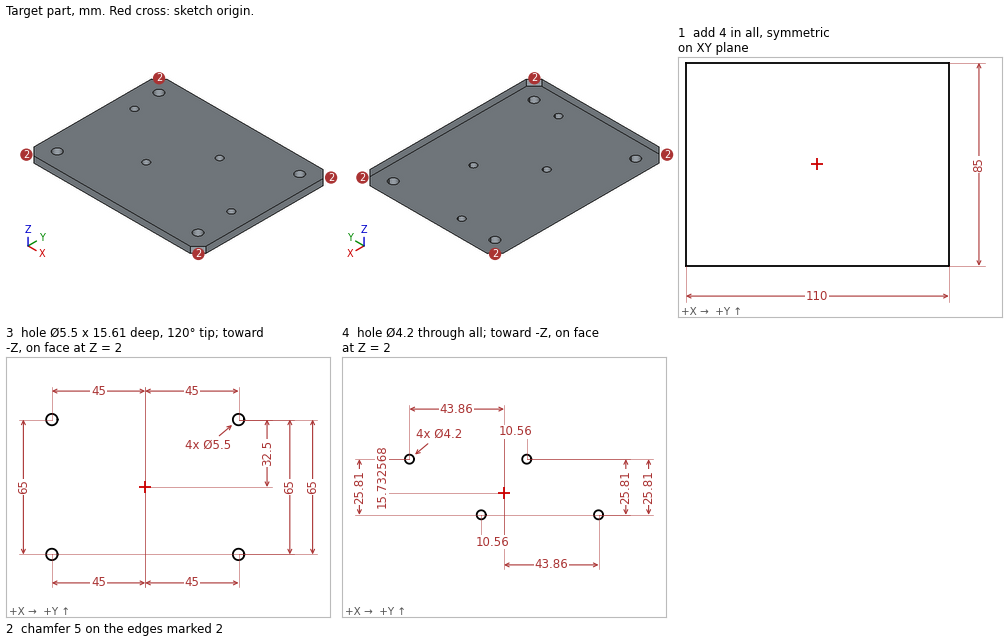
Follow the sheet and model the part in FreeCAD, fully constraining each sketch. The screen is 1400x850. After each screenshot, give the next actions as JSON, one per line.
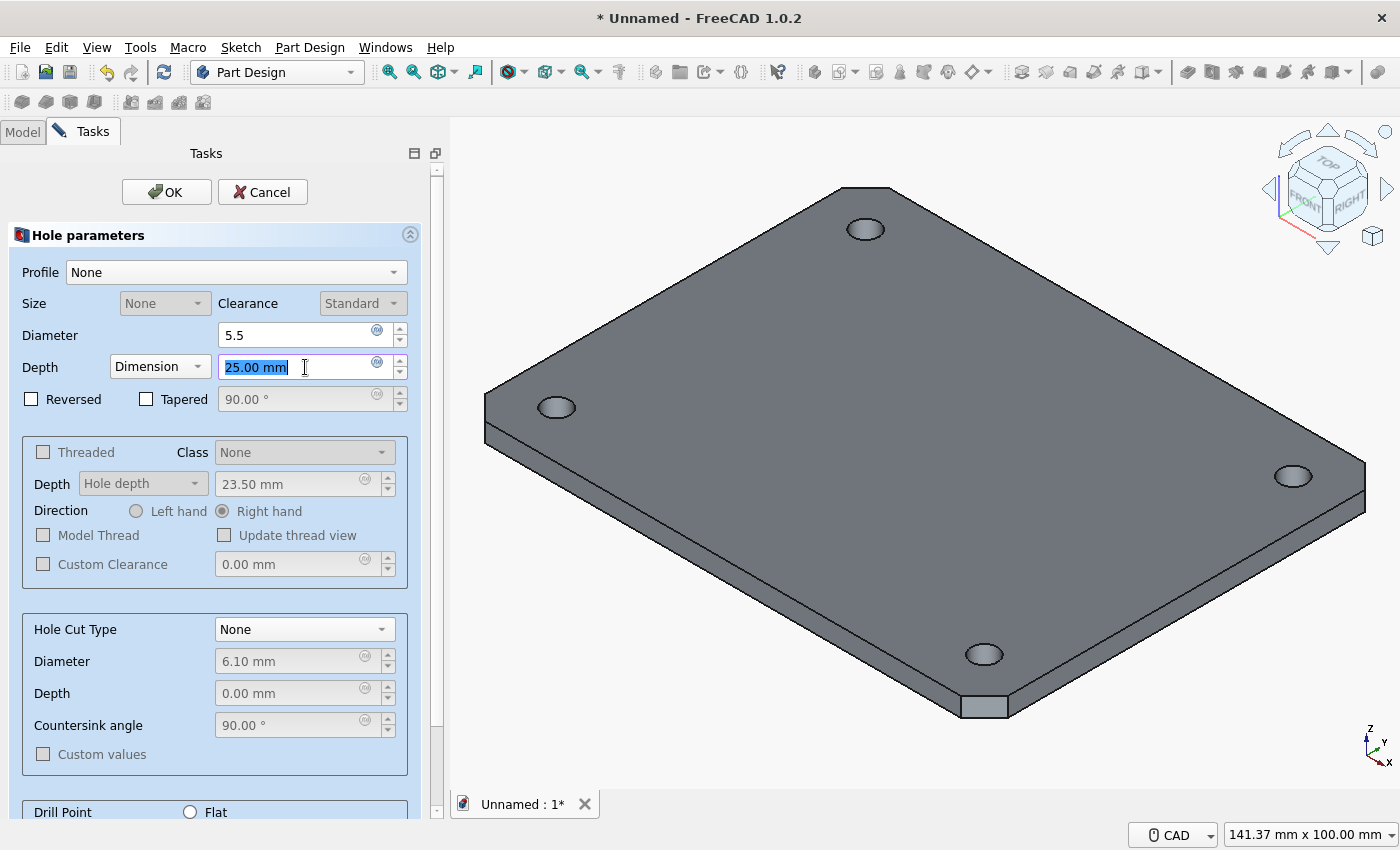
{"action": "type", "text": "15.61"}
{"action": "key", "text": "Tab"}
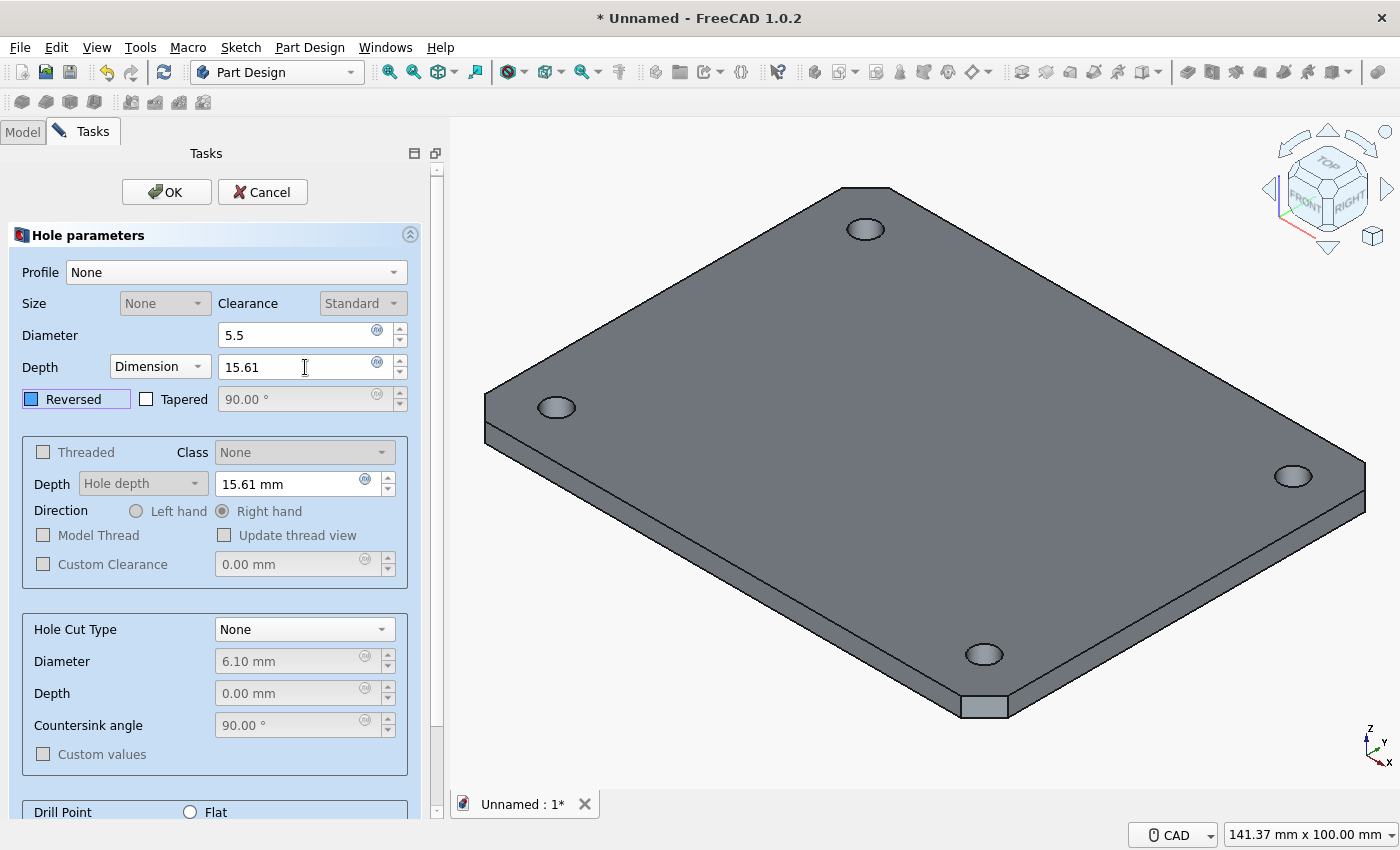
{"action": "scroll", "coordinate": [437, 490], "scroll_direction": "down", "scroll_amount": 2}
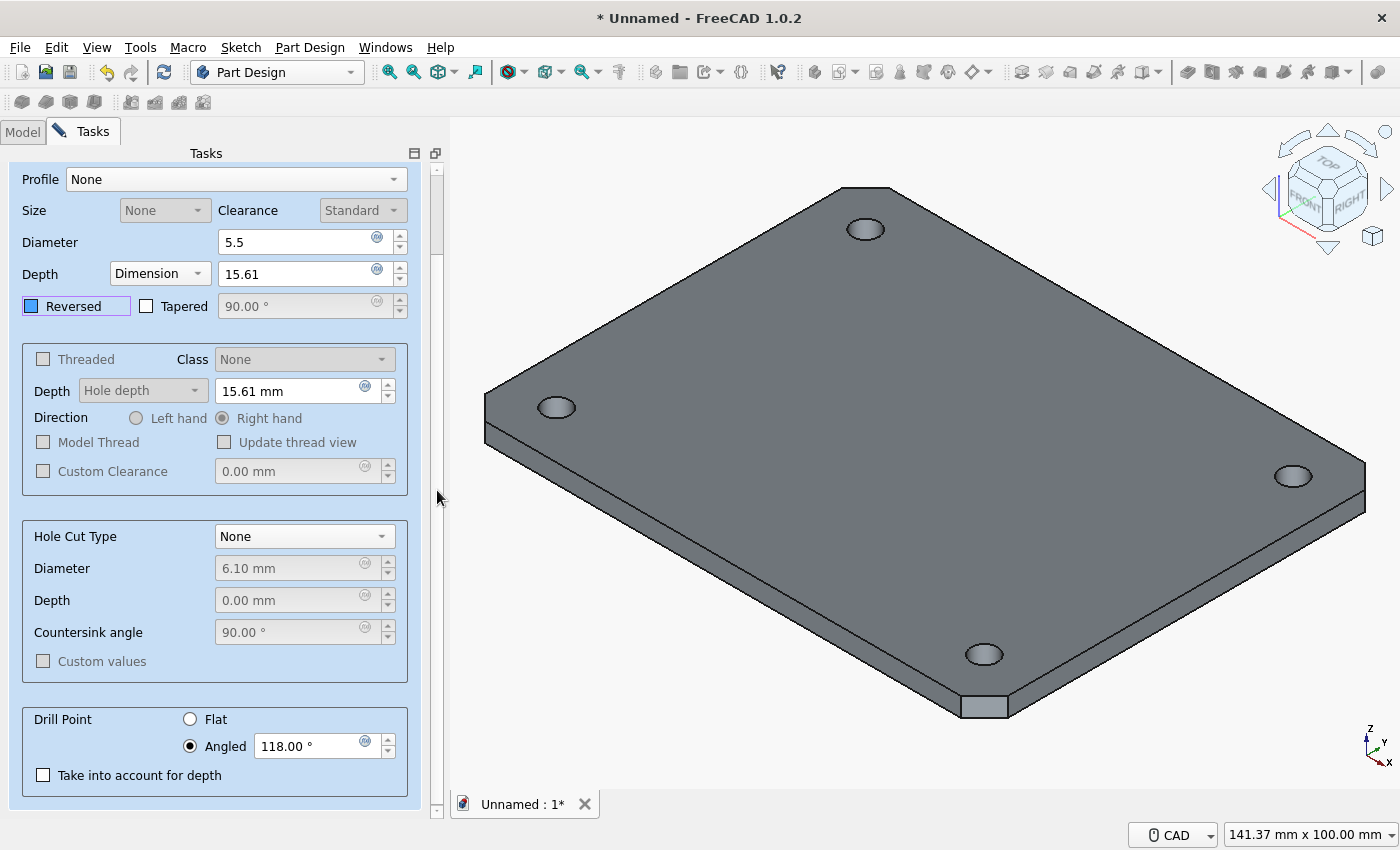
{"action": "triple_click", "coordinate": [317, 746]}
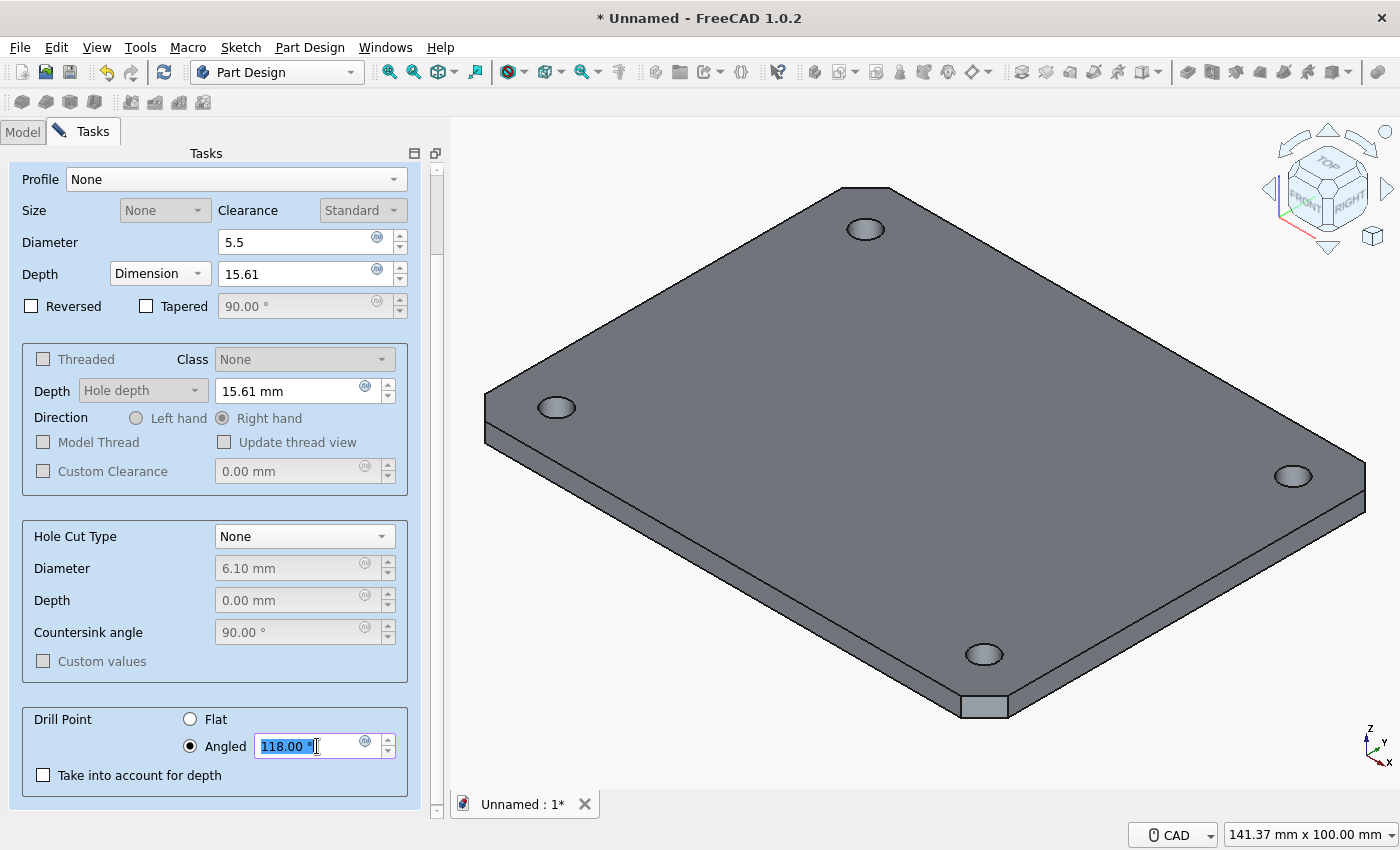
{"action": "type", "text": "120"}
{"action": "key", "text": "Tab"}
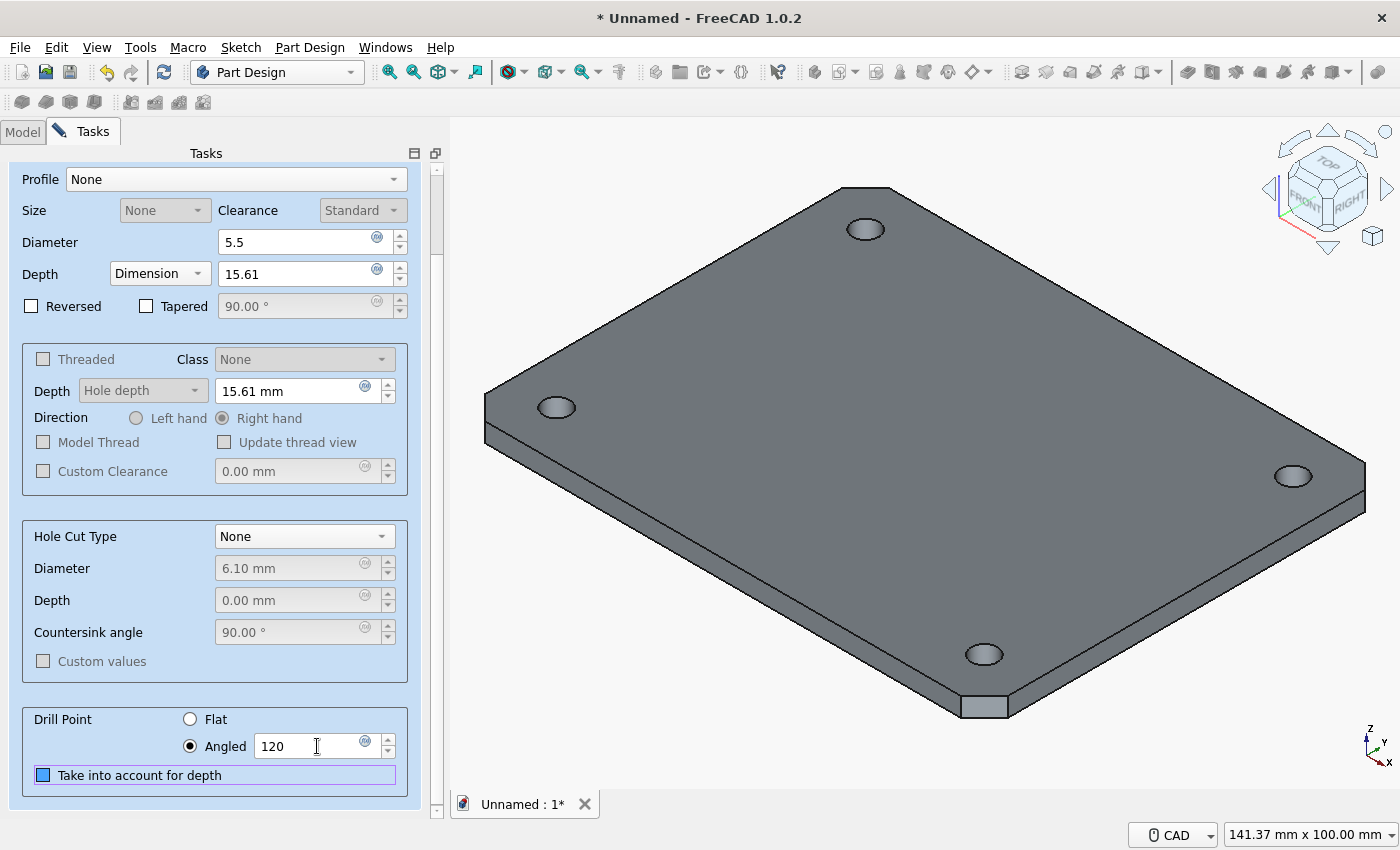
{"action": "scroll", "coordinate": [437, 490], "scroll_direction": "up", "scroll_amount": 3}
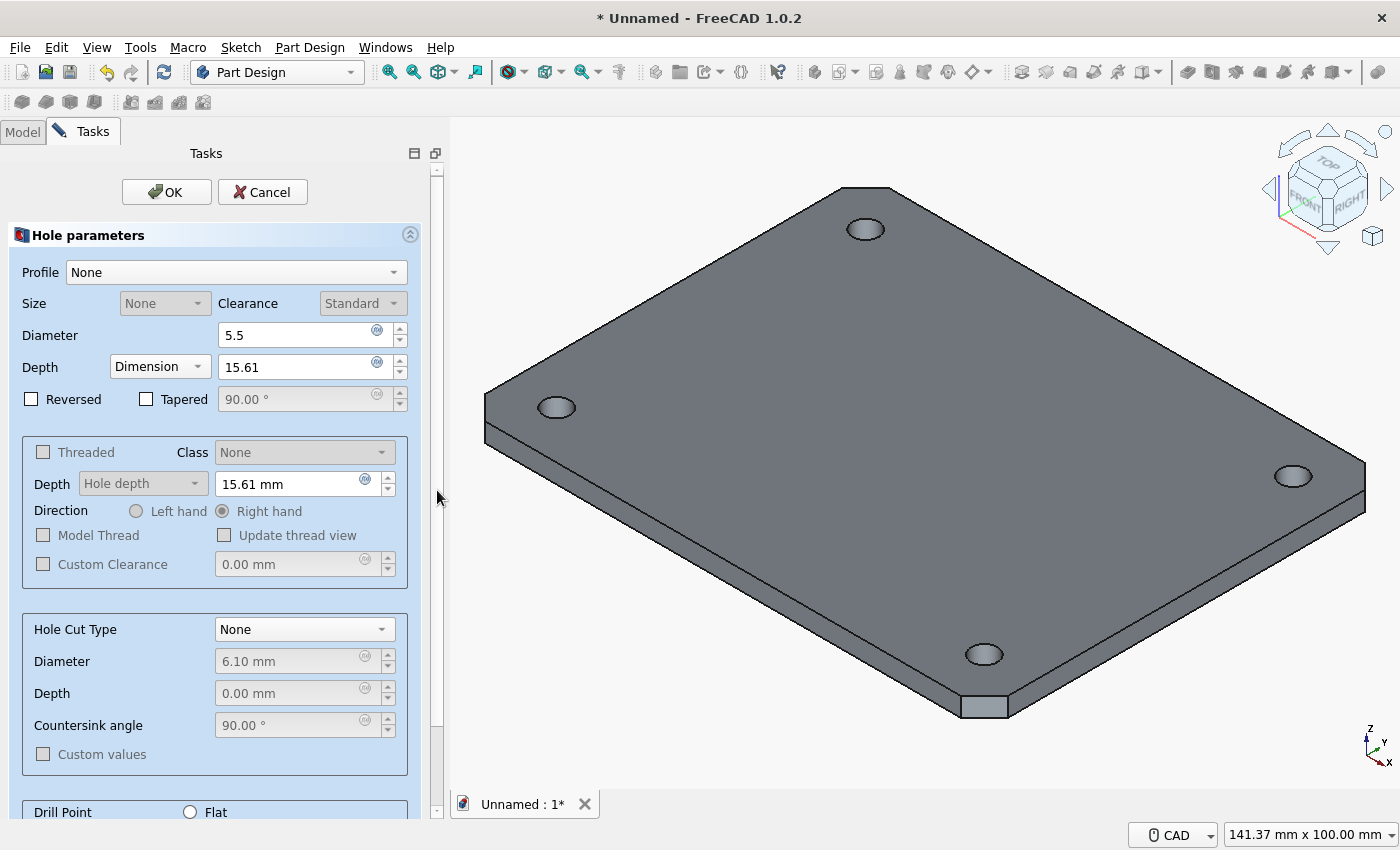
{"action": "left_click", "coordinate": [167, 192]}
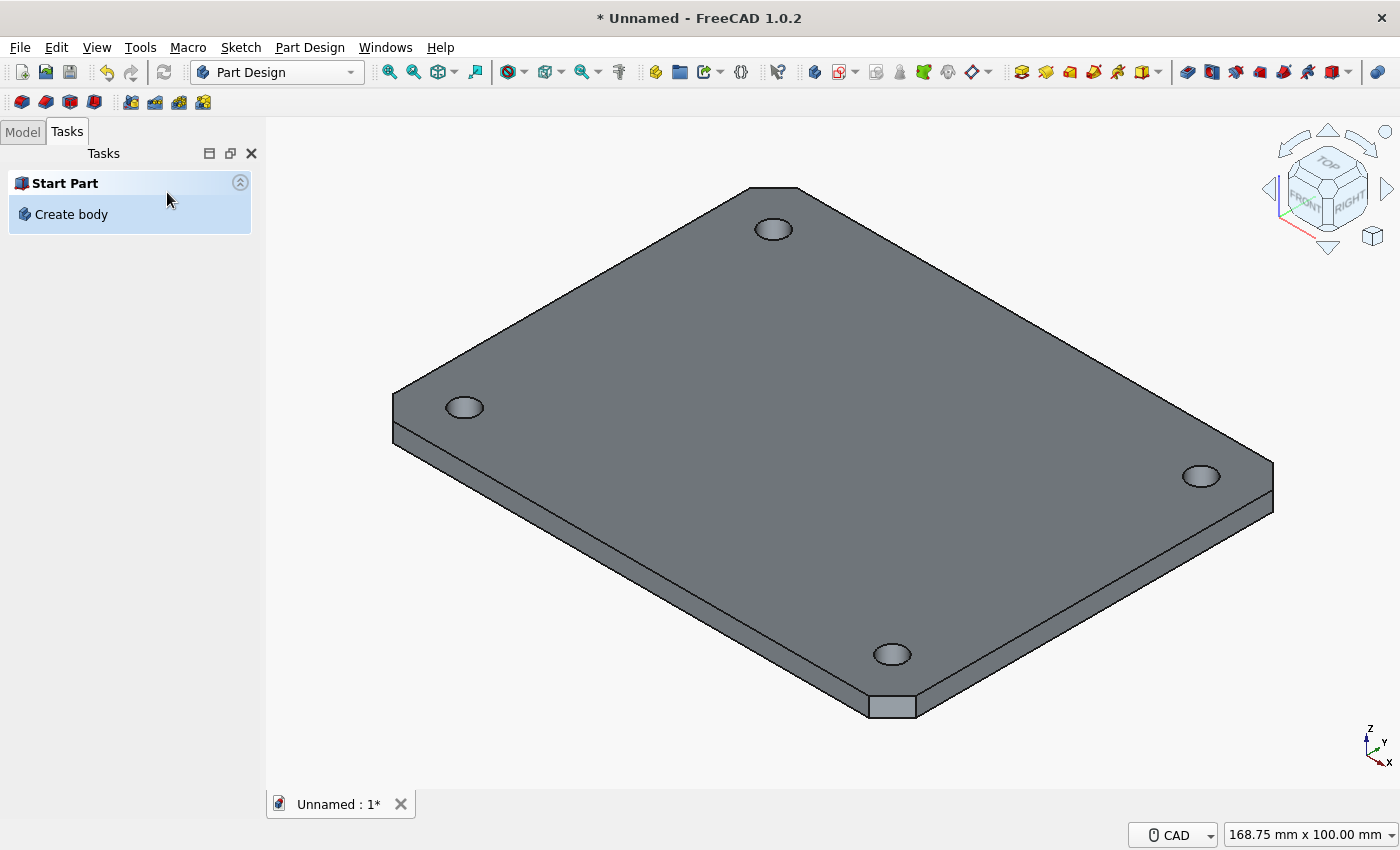
{"action": "left_click", "coordinate": [833, 441]}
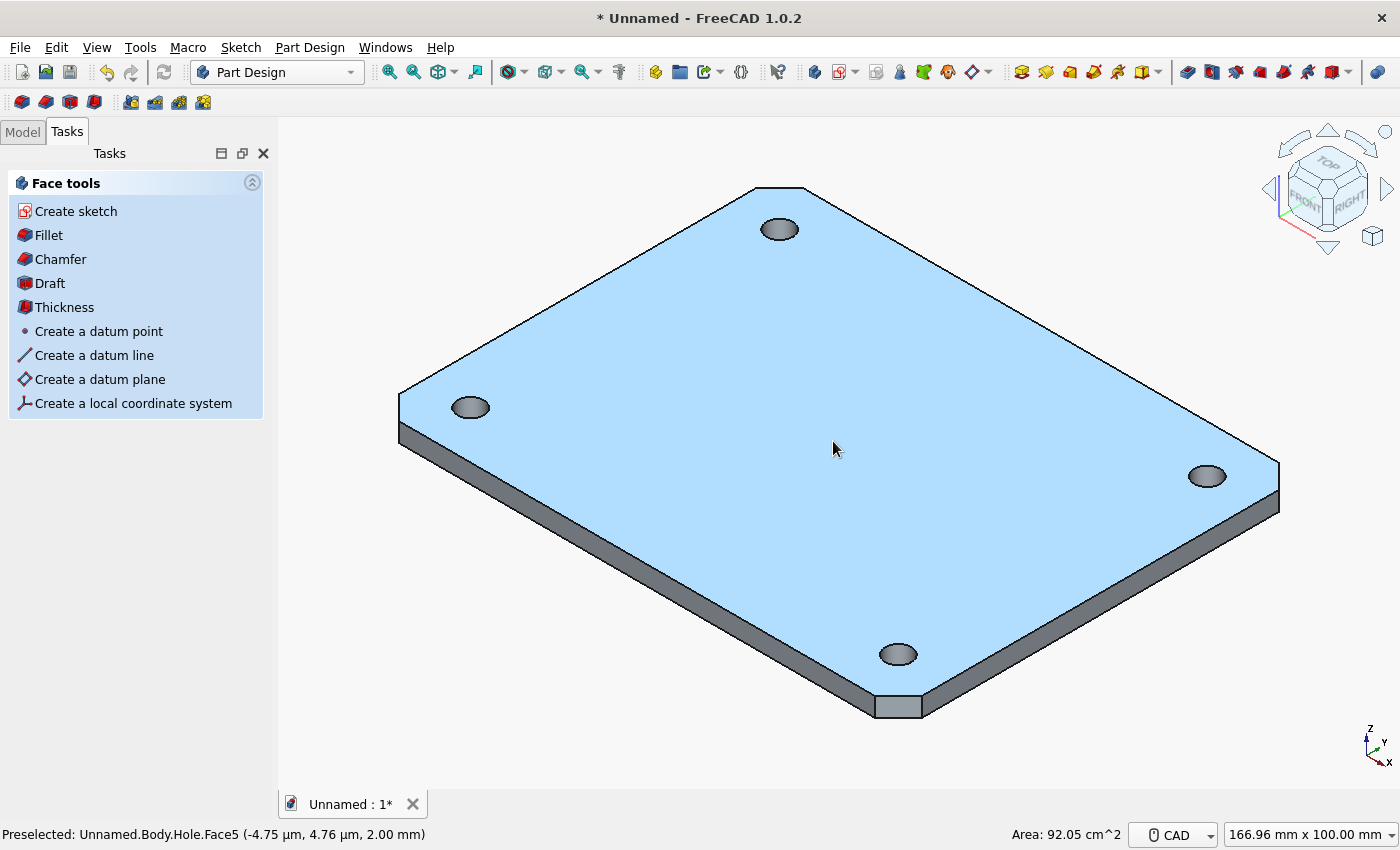
{"action": "left_click", "coordinate": [840, 72]}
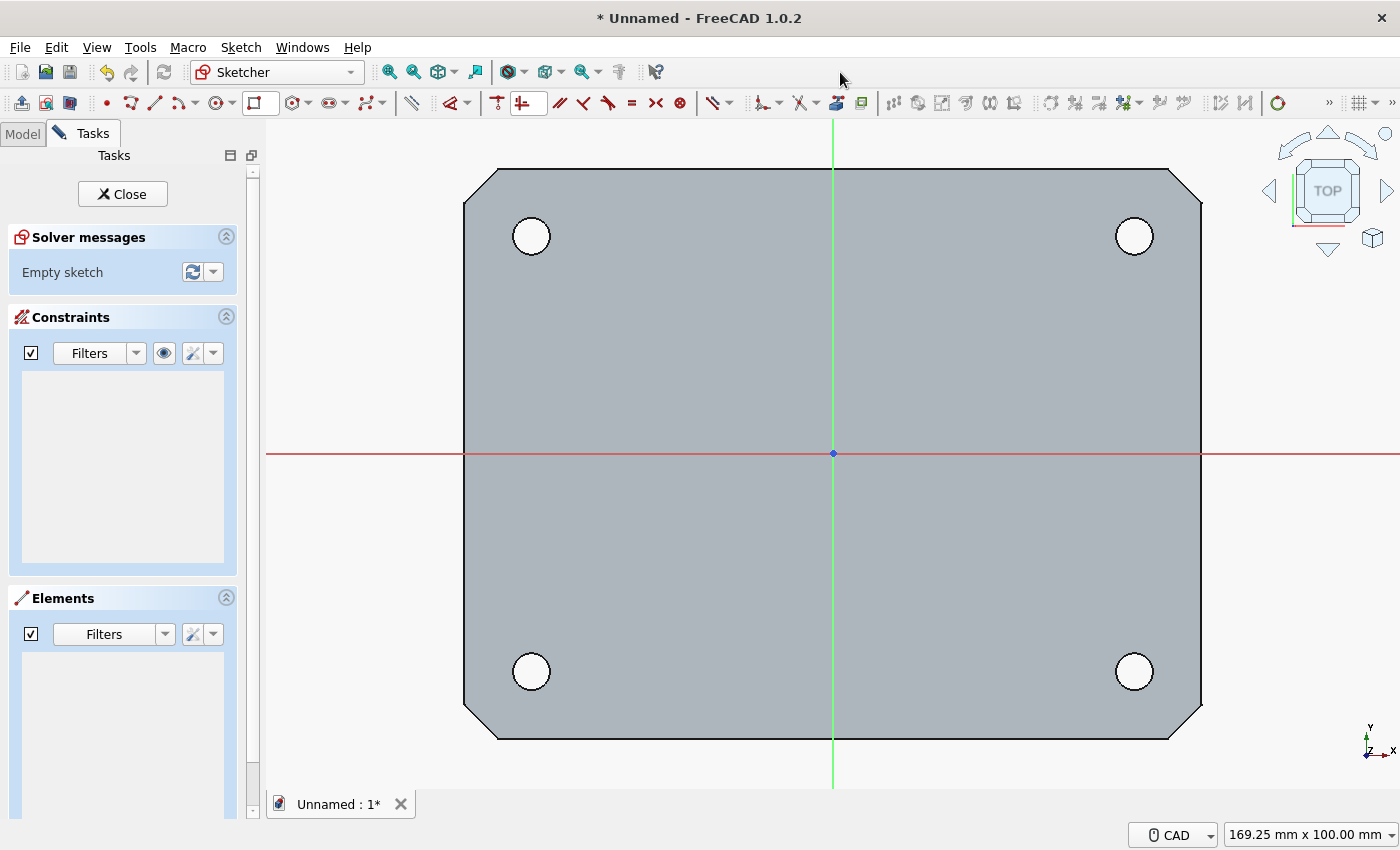
{"action": "left_click", "coordinate": [216, 104]}